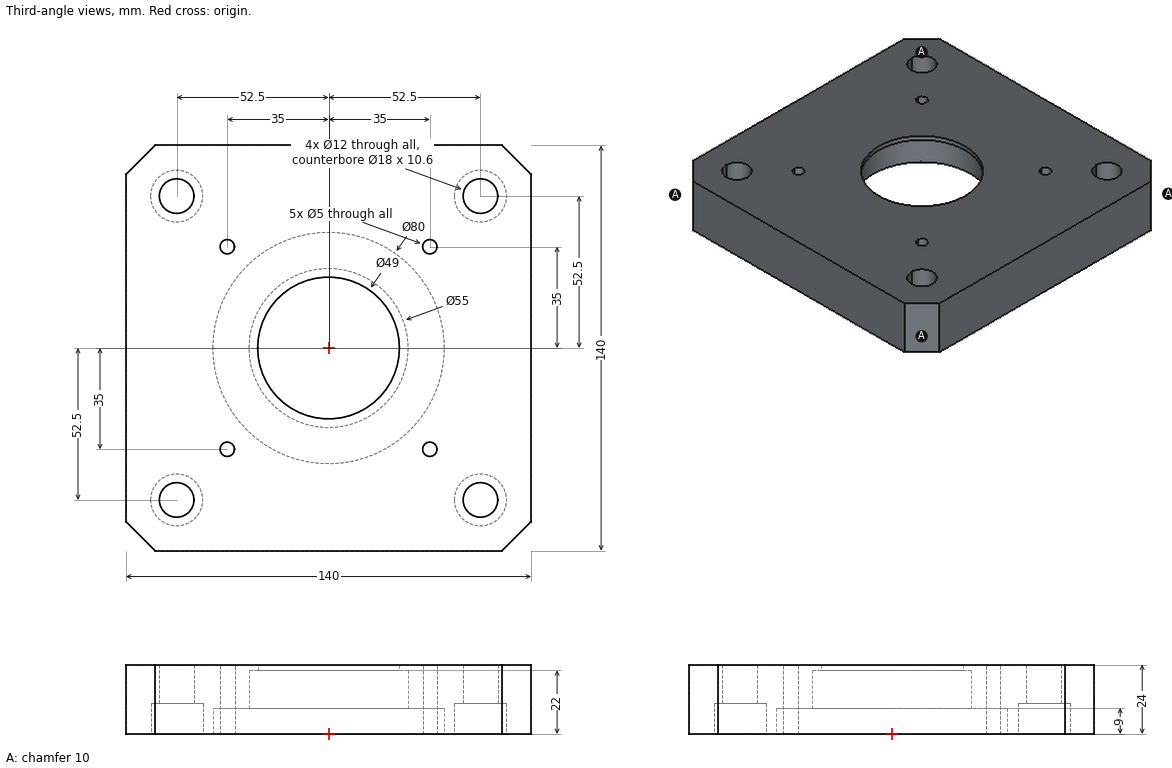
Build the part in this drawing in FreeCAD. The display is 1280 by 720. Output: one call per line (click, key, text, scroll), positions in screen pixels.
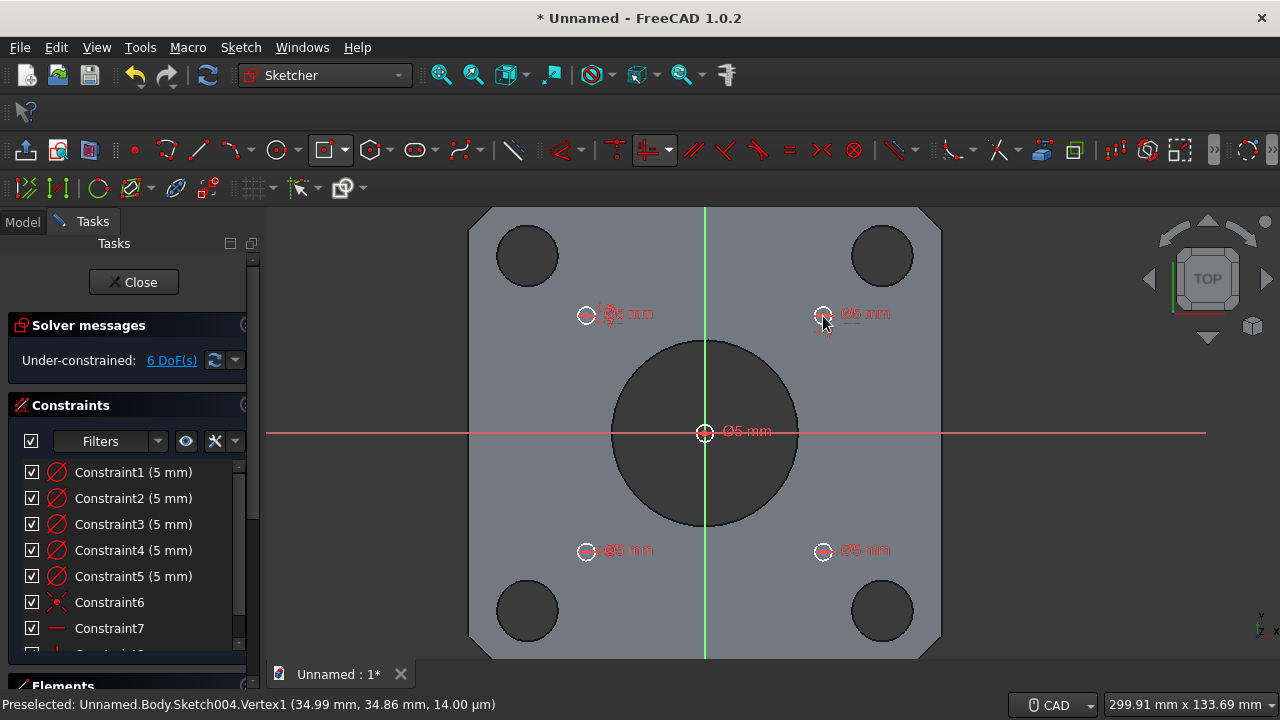
click(823, 552)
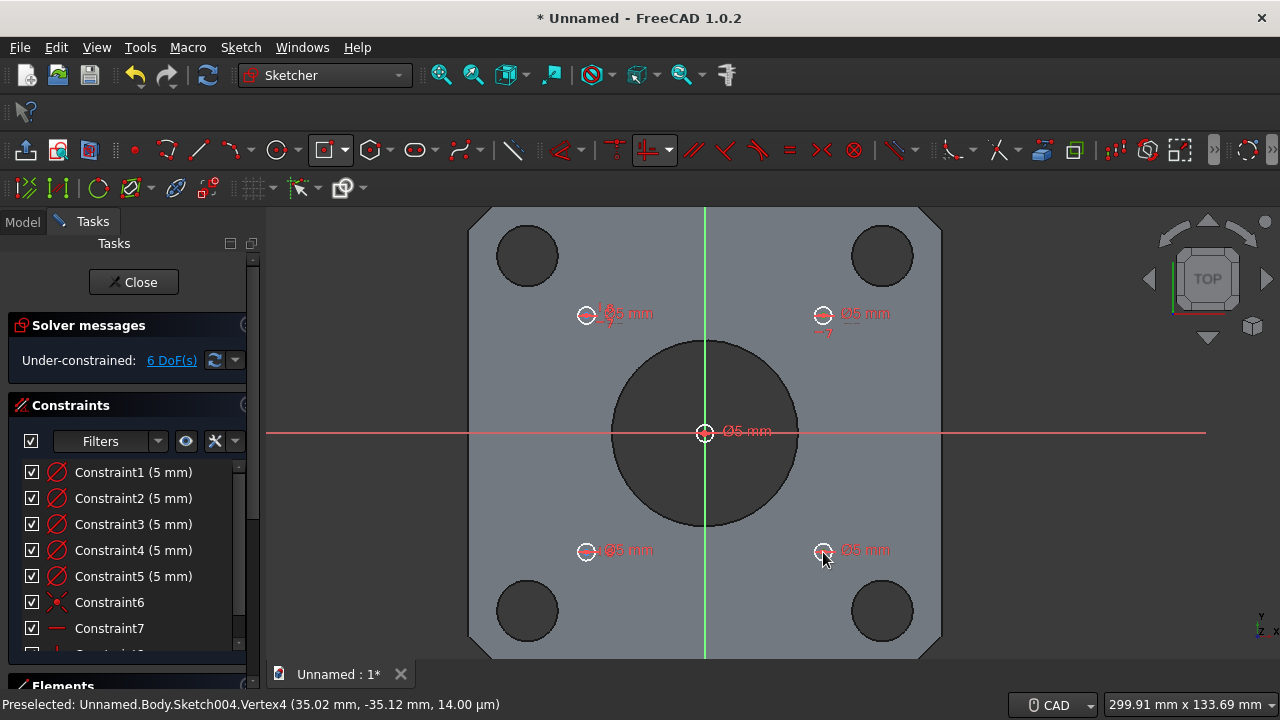
click(672, 150)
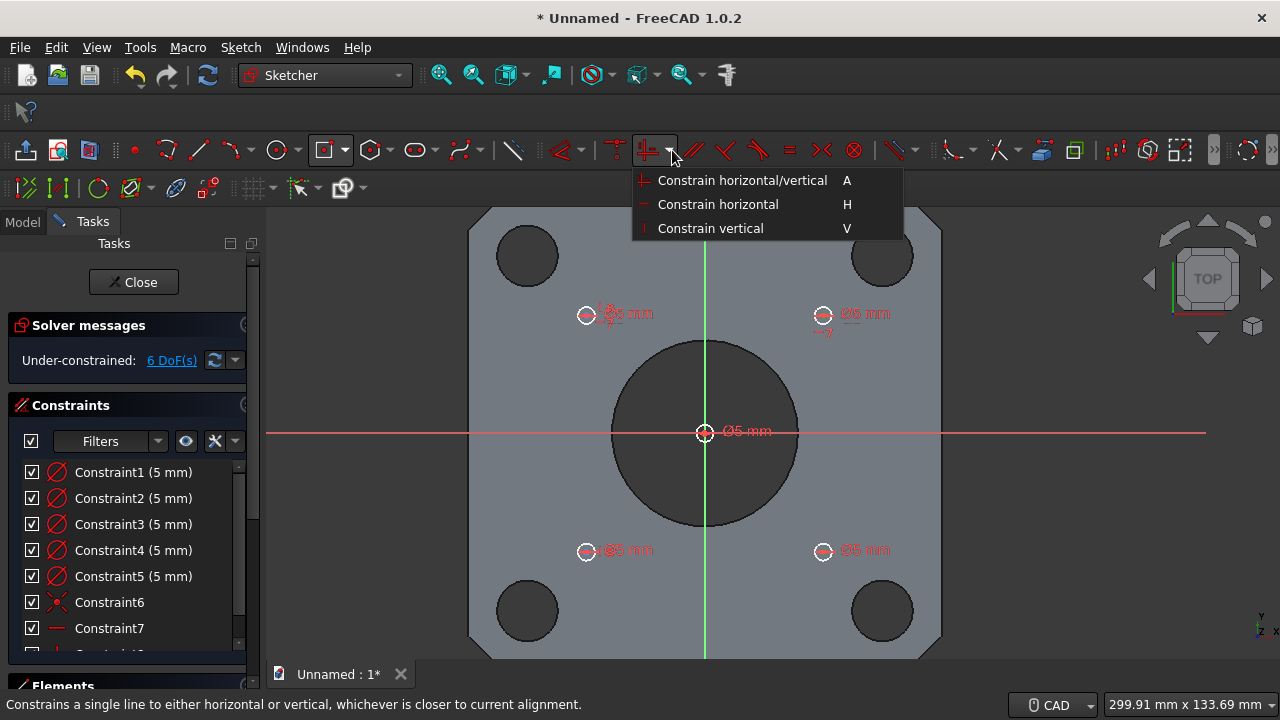
click(768, 228)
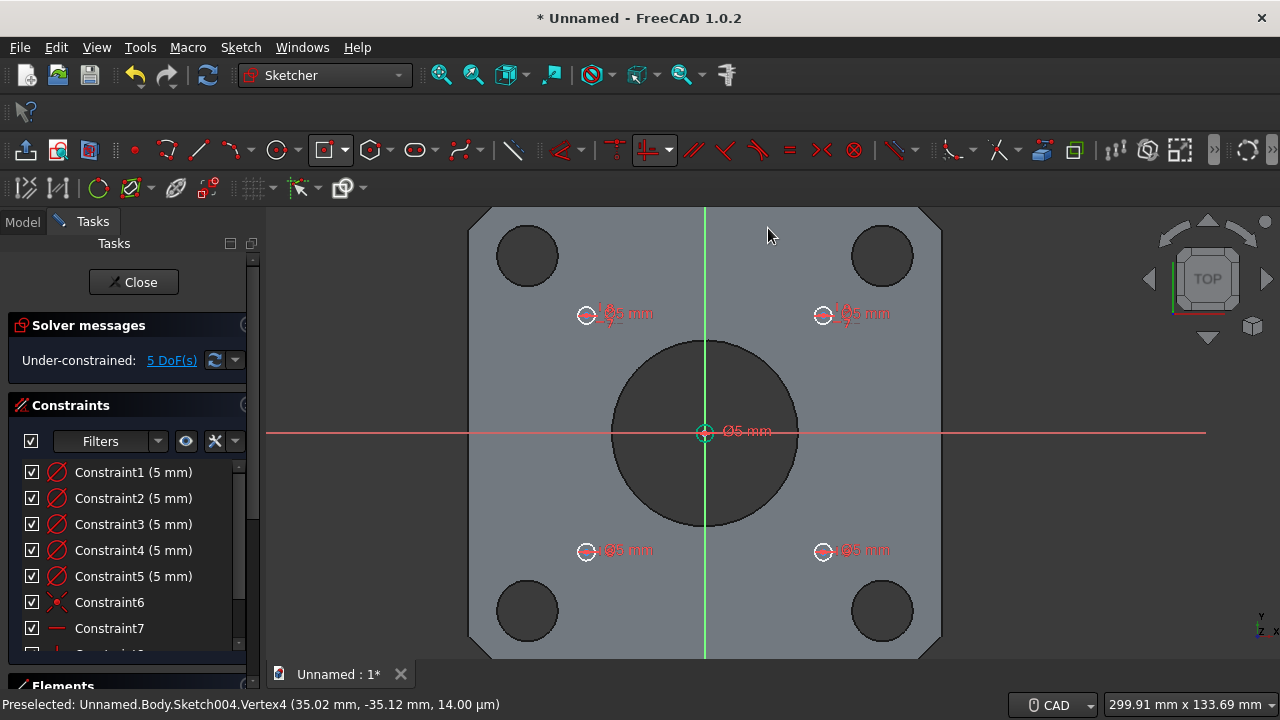
click(586, 552)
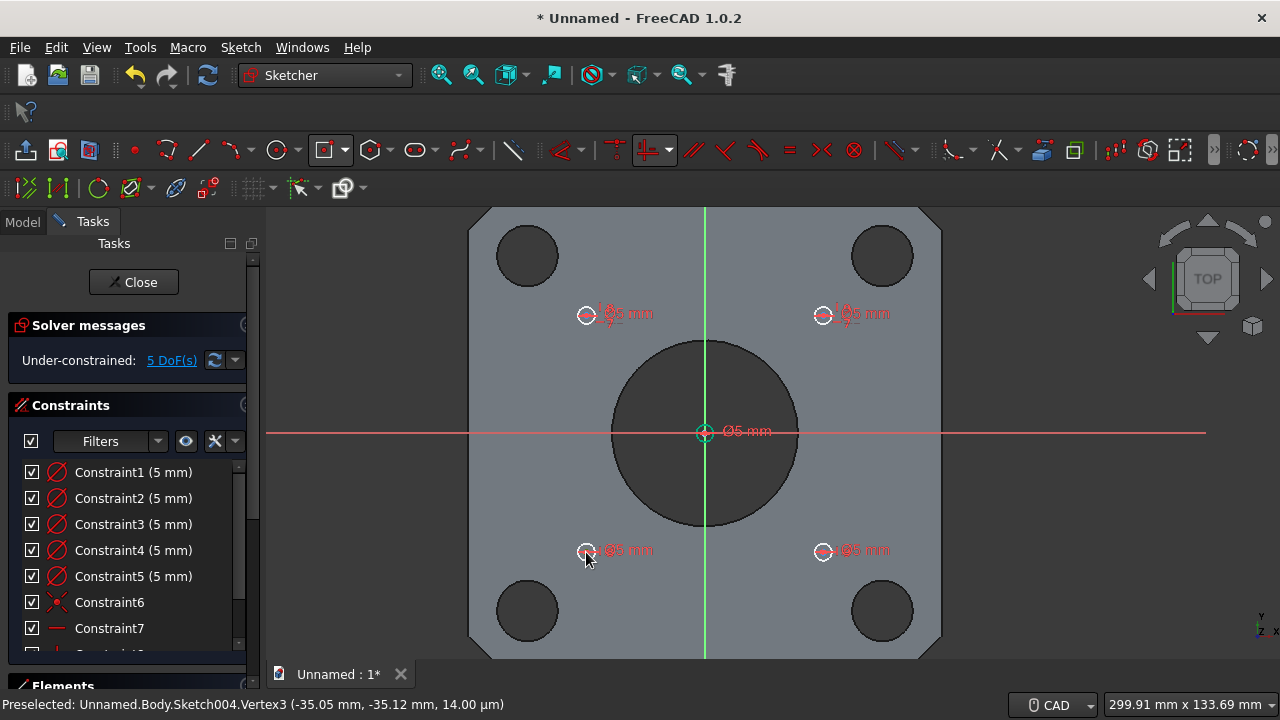
click(823, 552)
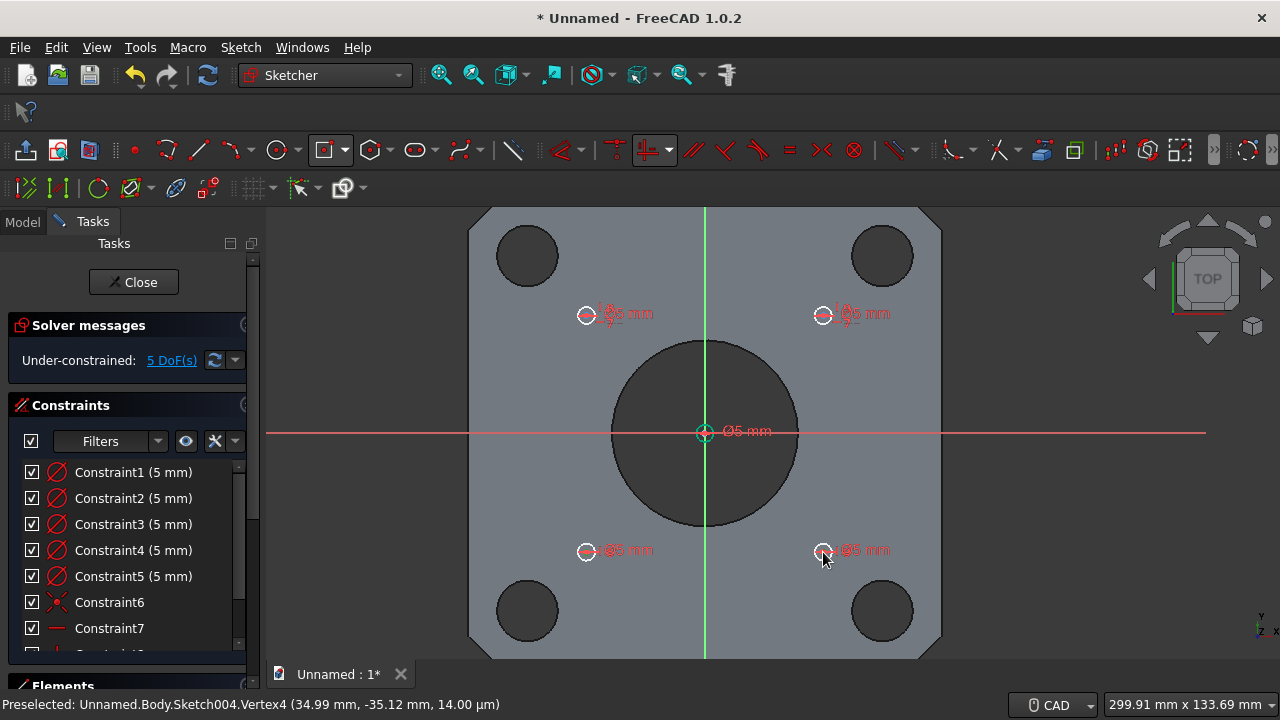
key(h)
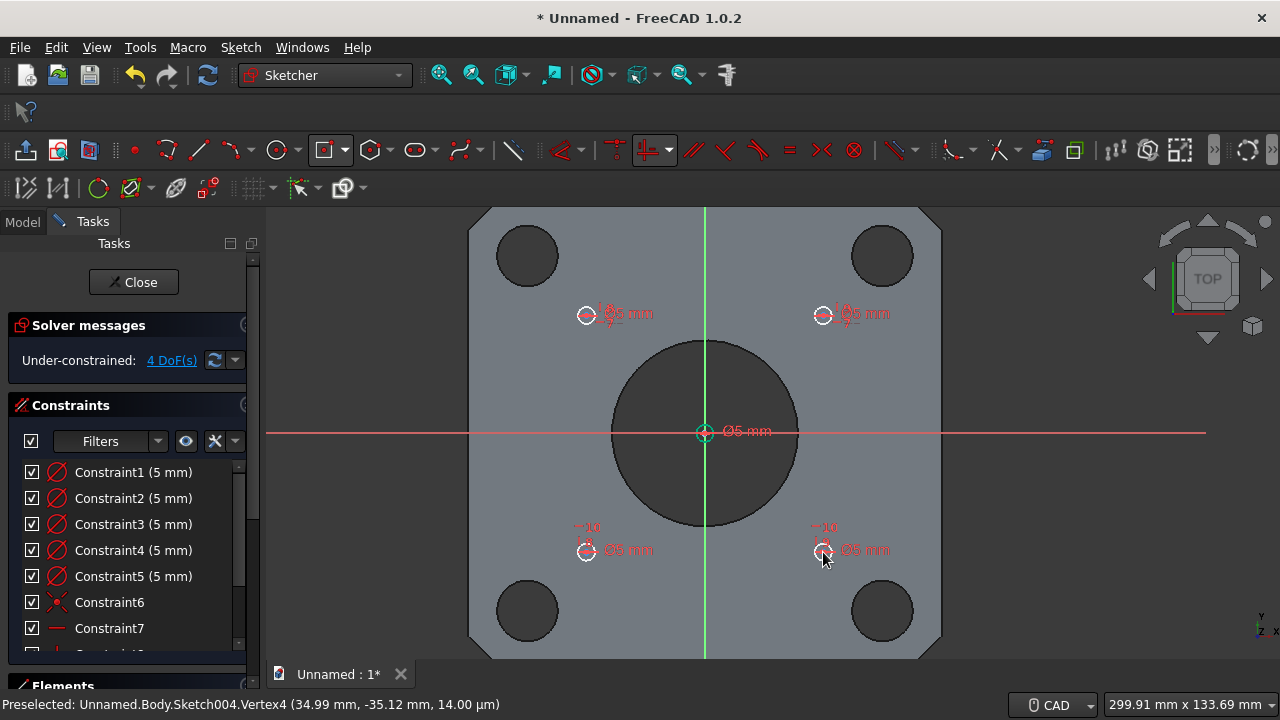
click(560, 150)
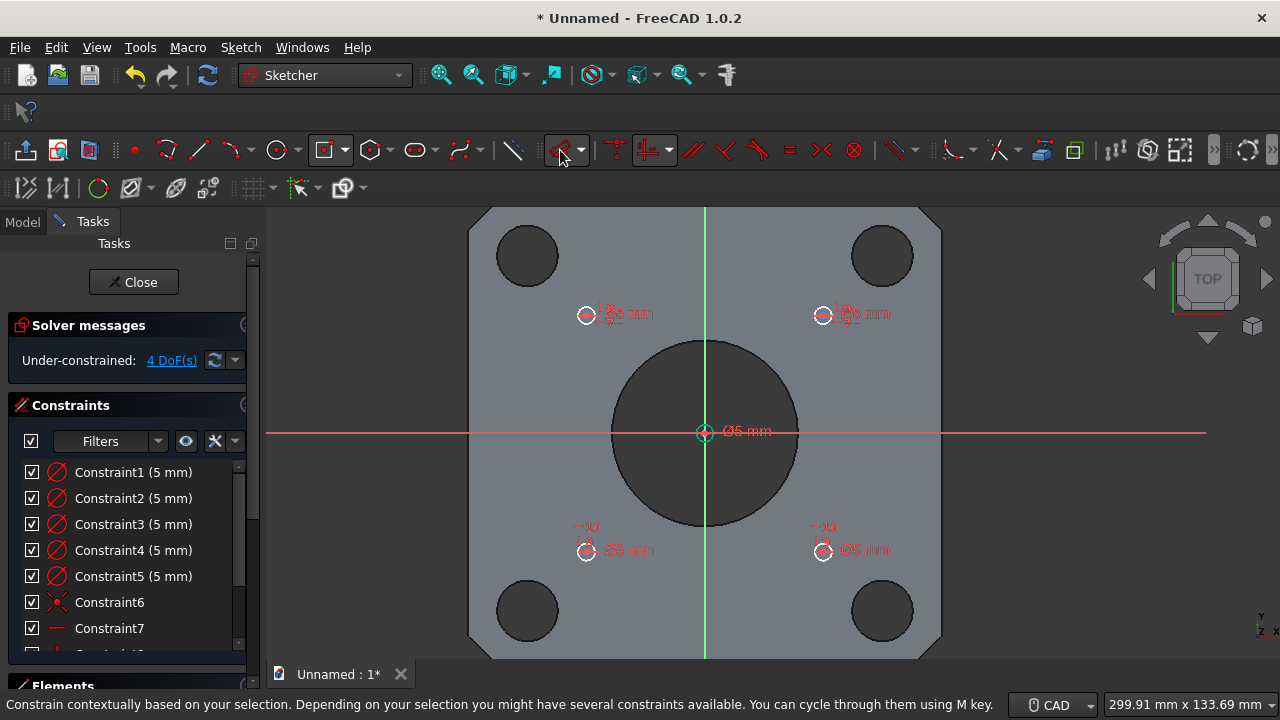
click(823, 316)
click(764, 282)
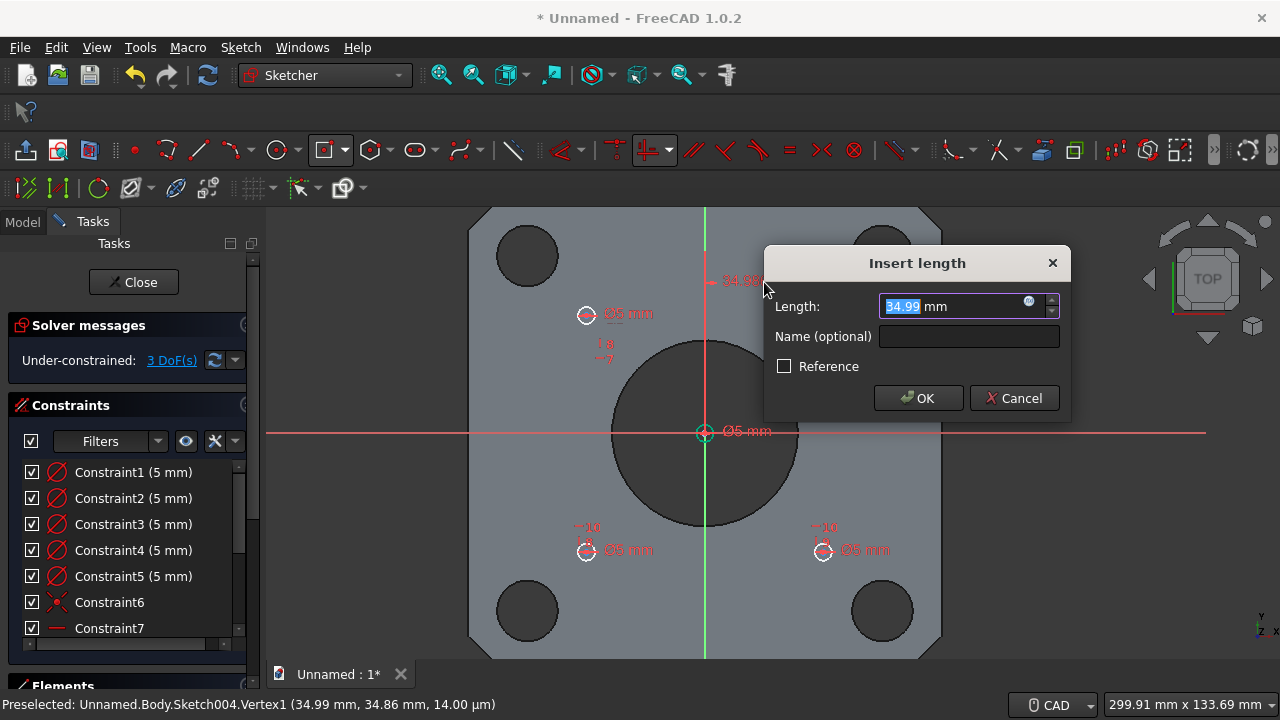
text(35)
key(Return)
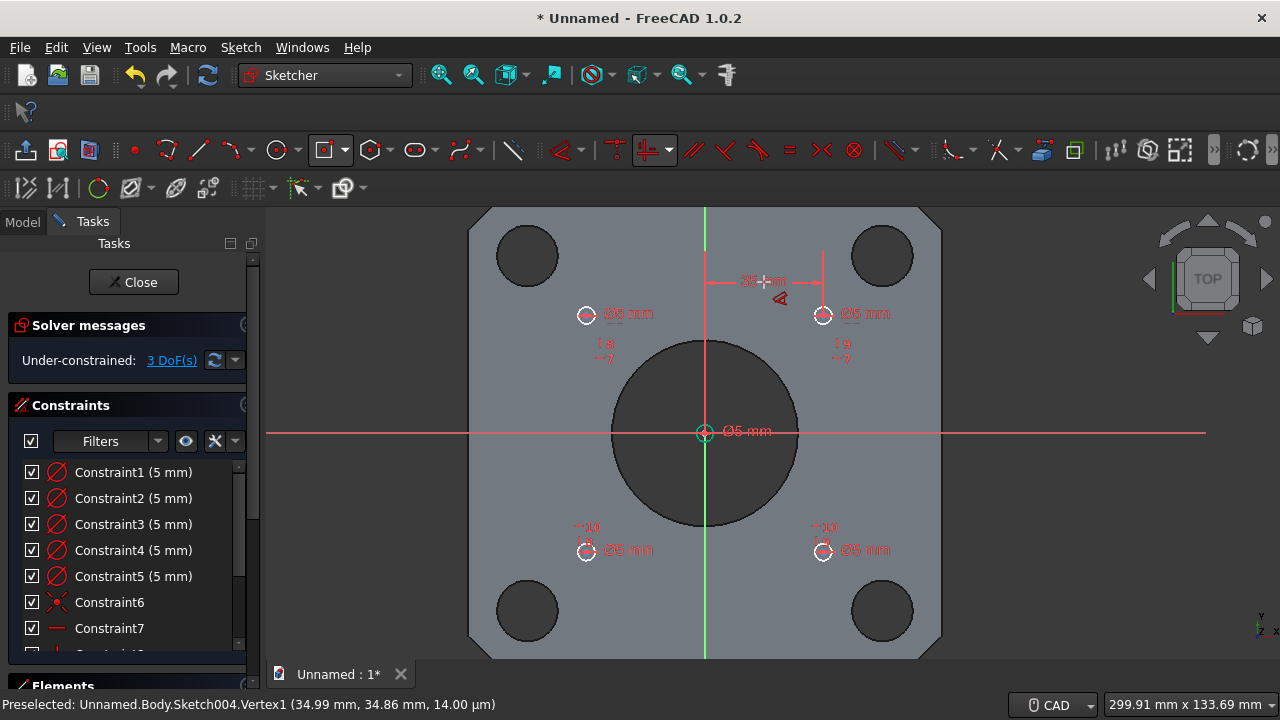
click(823, 316)
click(857, 374)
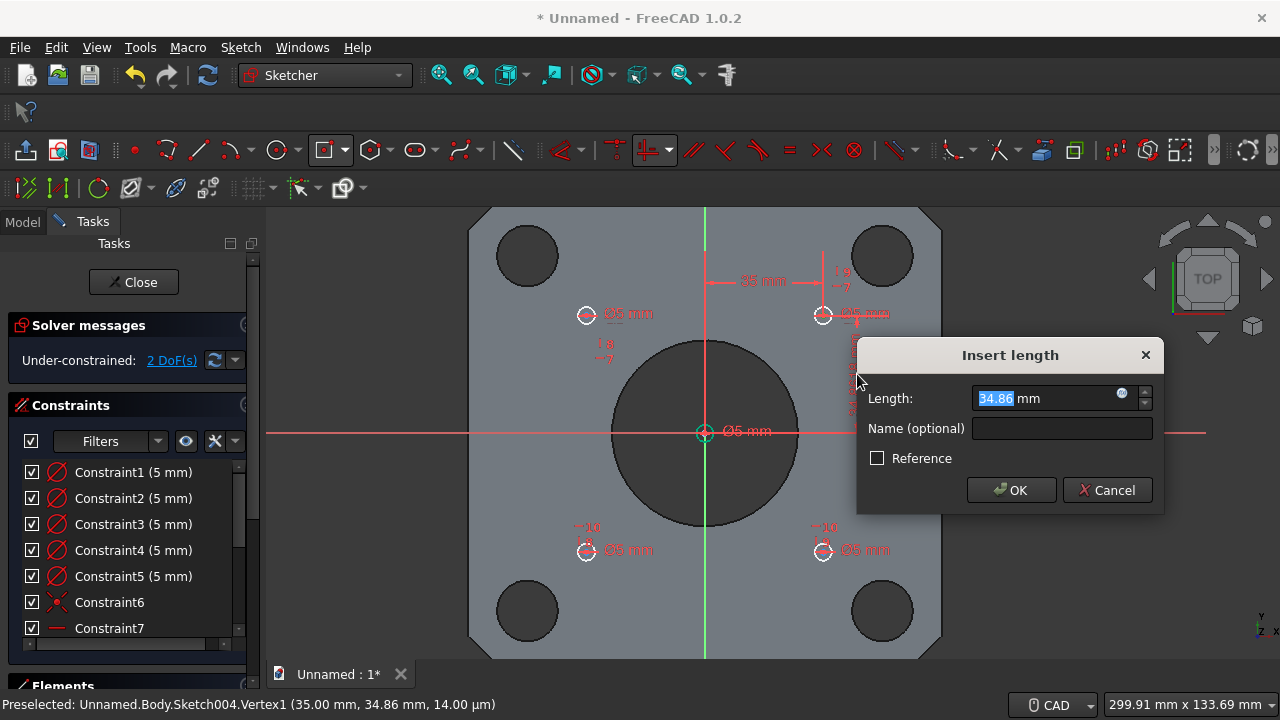
text(35)
key(Return)